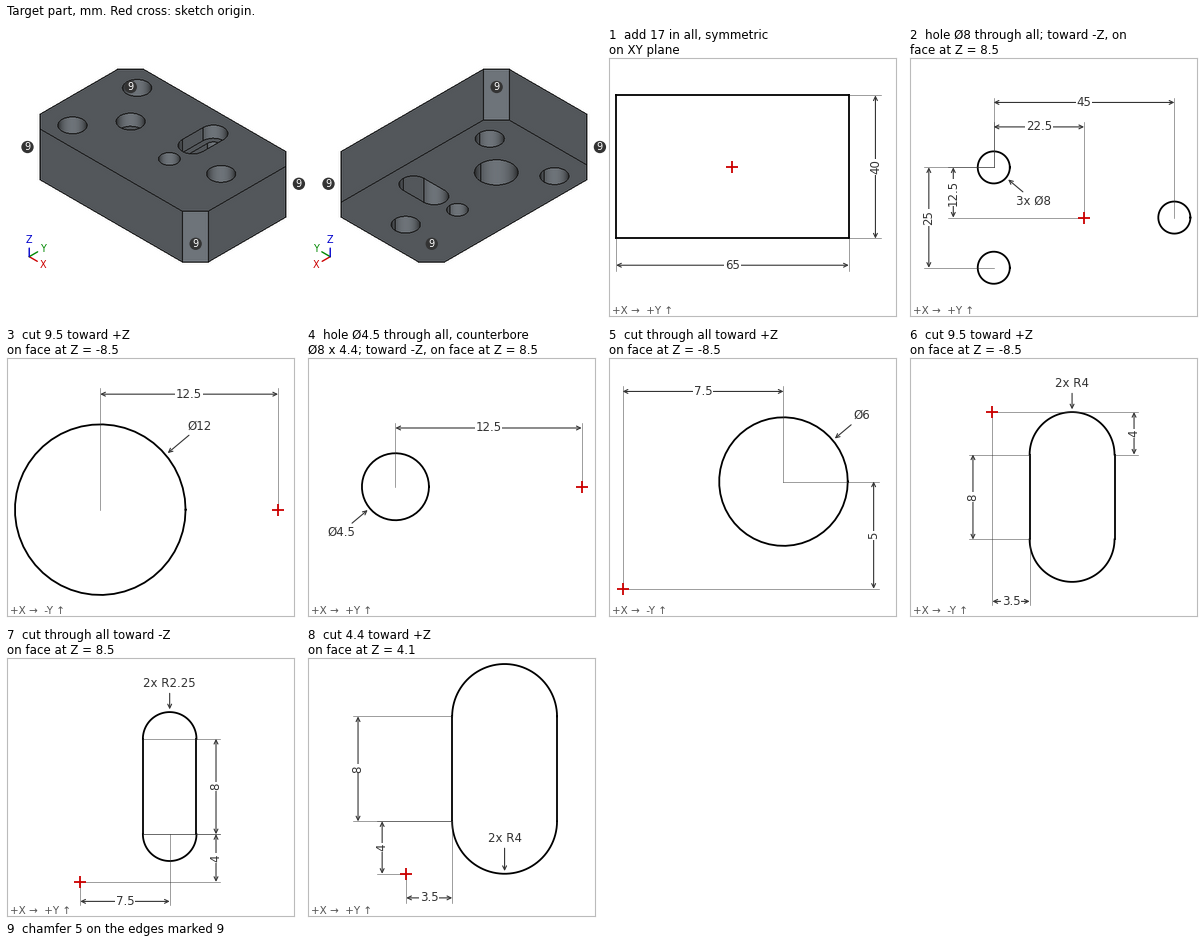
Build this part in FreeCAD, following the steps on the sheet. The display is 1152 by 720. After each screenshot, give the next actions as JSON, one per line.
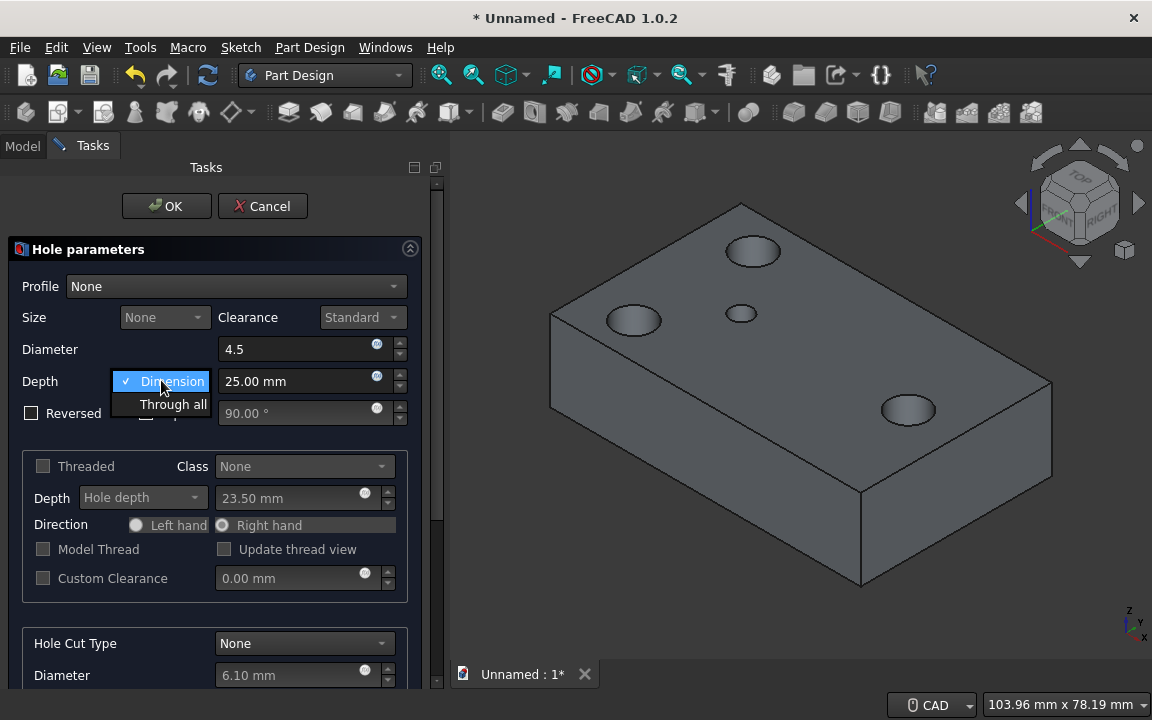
{"action": "left_click", "coordinate": [160, 404]}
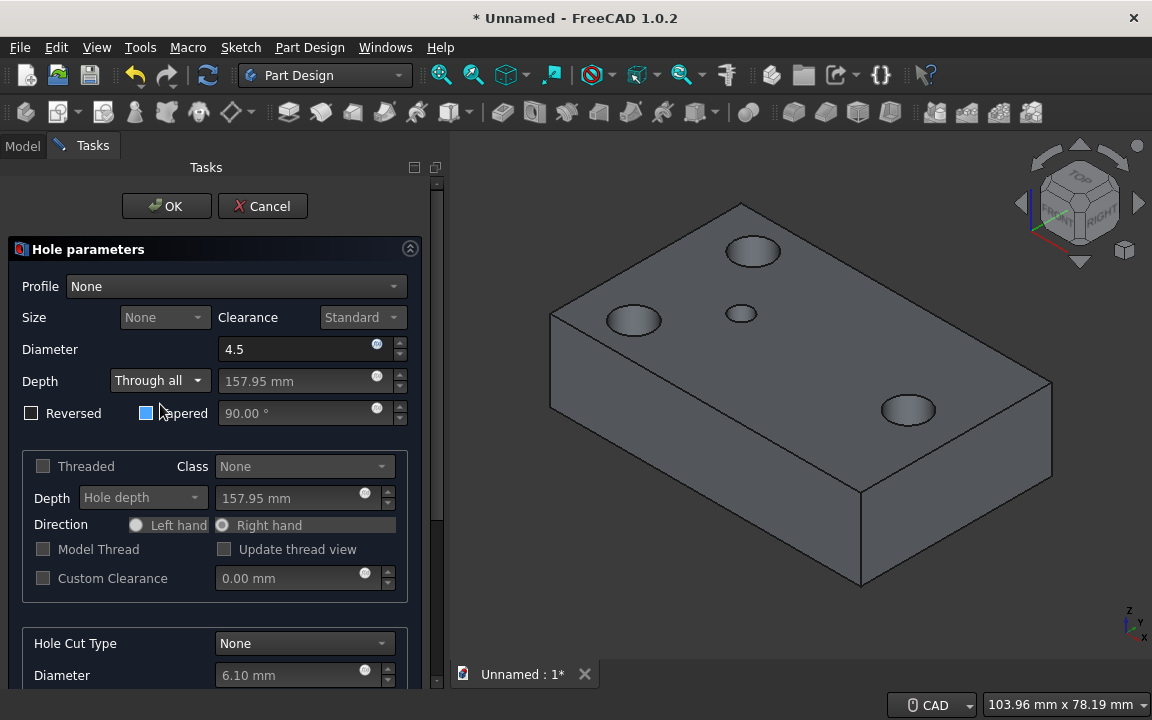
{"action": "left_click", "coordinate": [306, 644]}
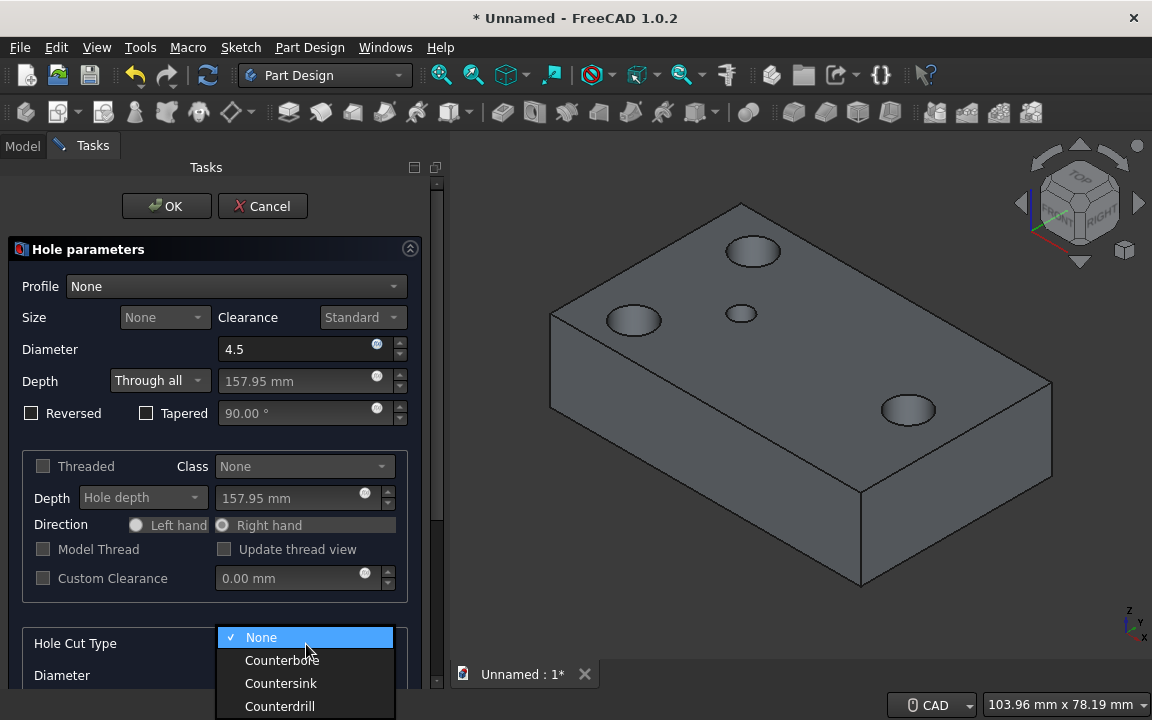
{"action": "left_click", "coordinate": [304, 660]}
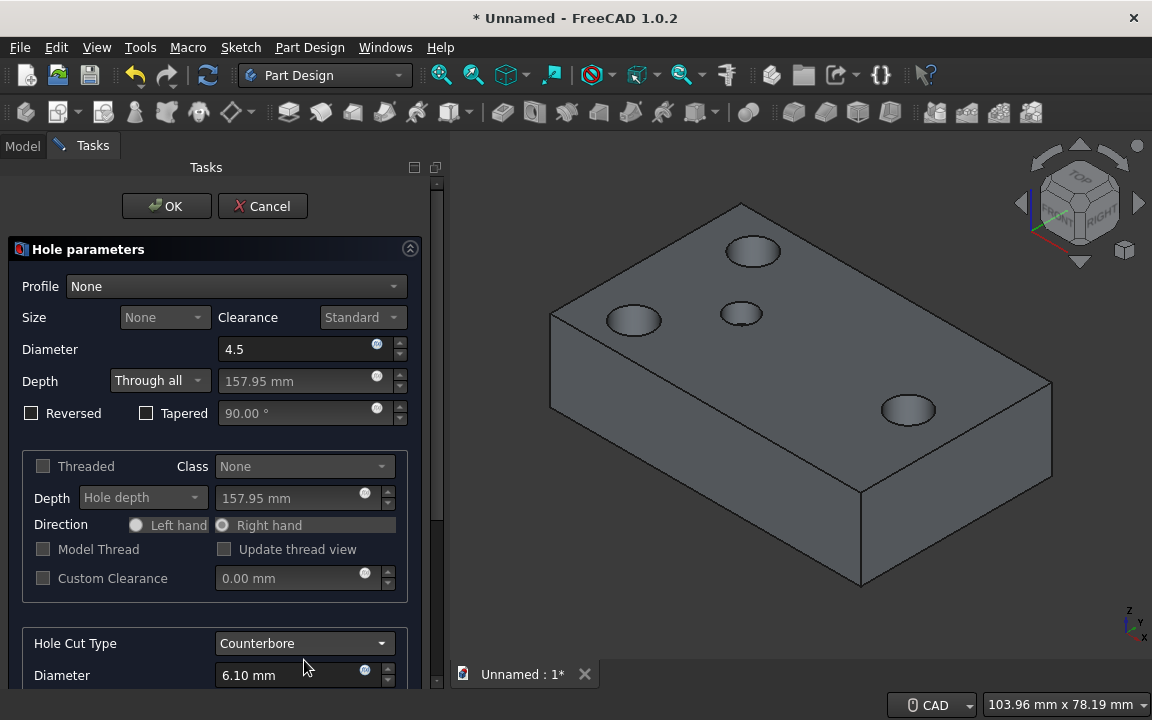
{"action": "triple_click", "coordinate": [298, 675]}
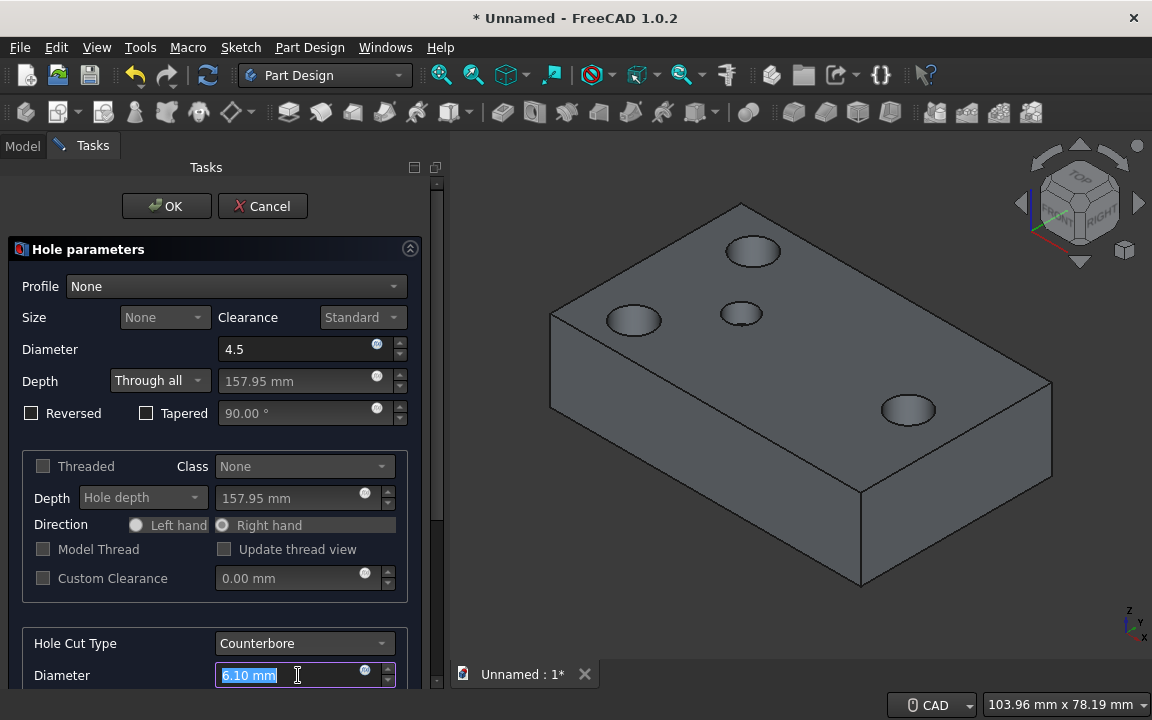
{"action": "type", "text": "8"}
{"action": "key", "text": "Tab"}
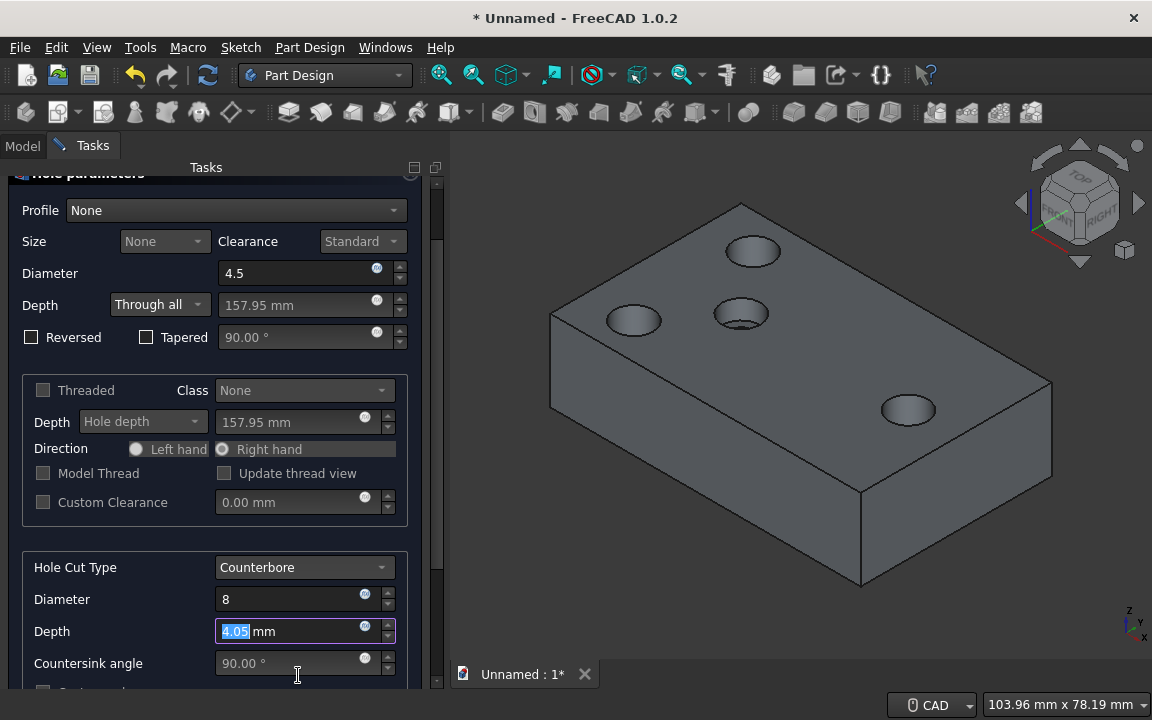
{"action": "type", "text": "4.4"}
{"action": "key", "text": "Tab"}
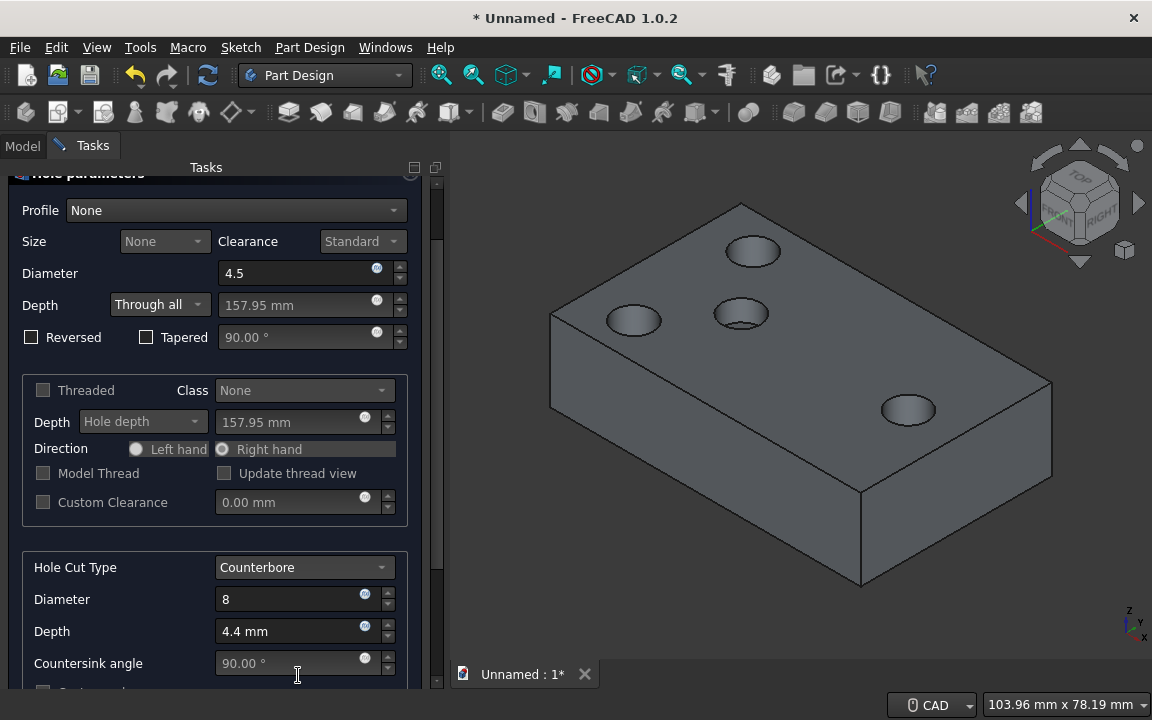
{"action": "scroll", "coordinate": [437, 432], "scroll_direction": "up", "scroll_amount": 3}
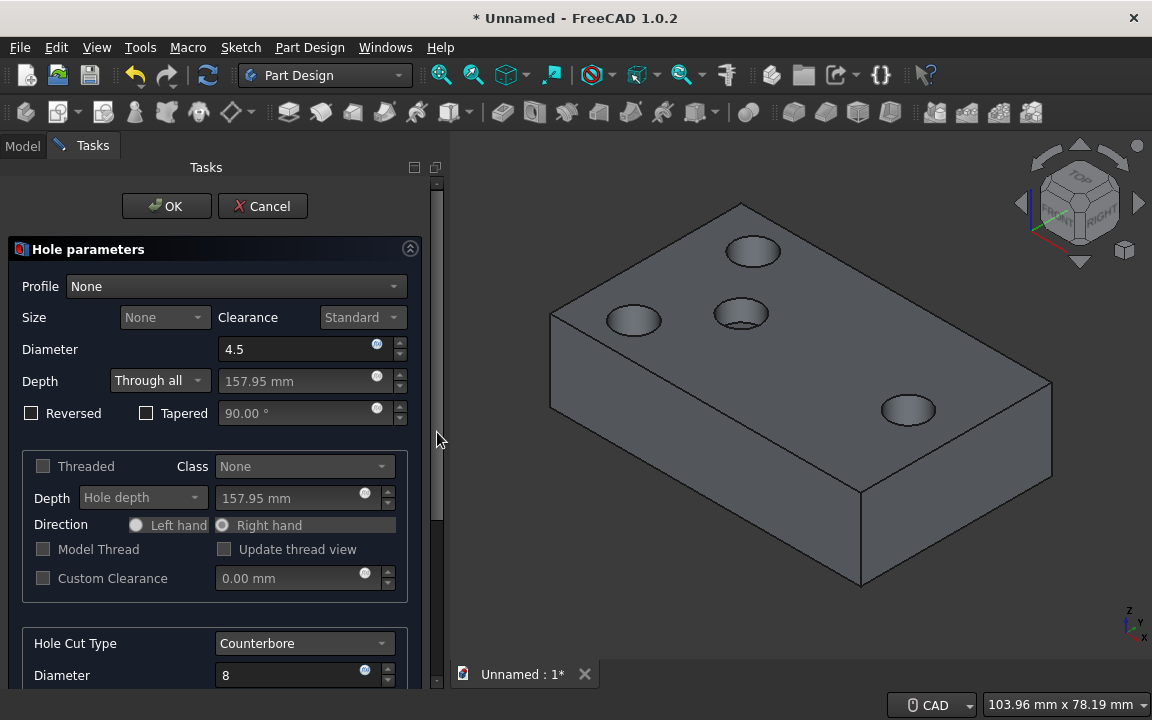
{"action": "left_click", "coordinate": [167, 206]}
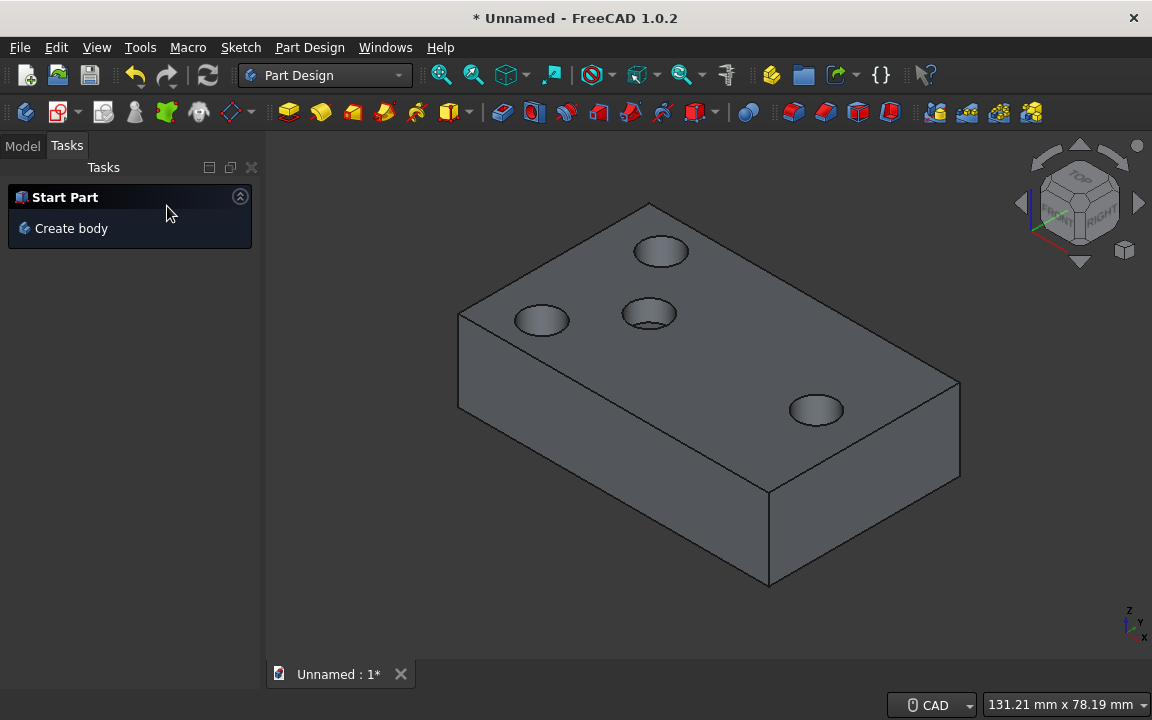
{"action": "key", "text": "5"}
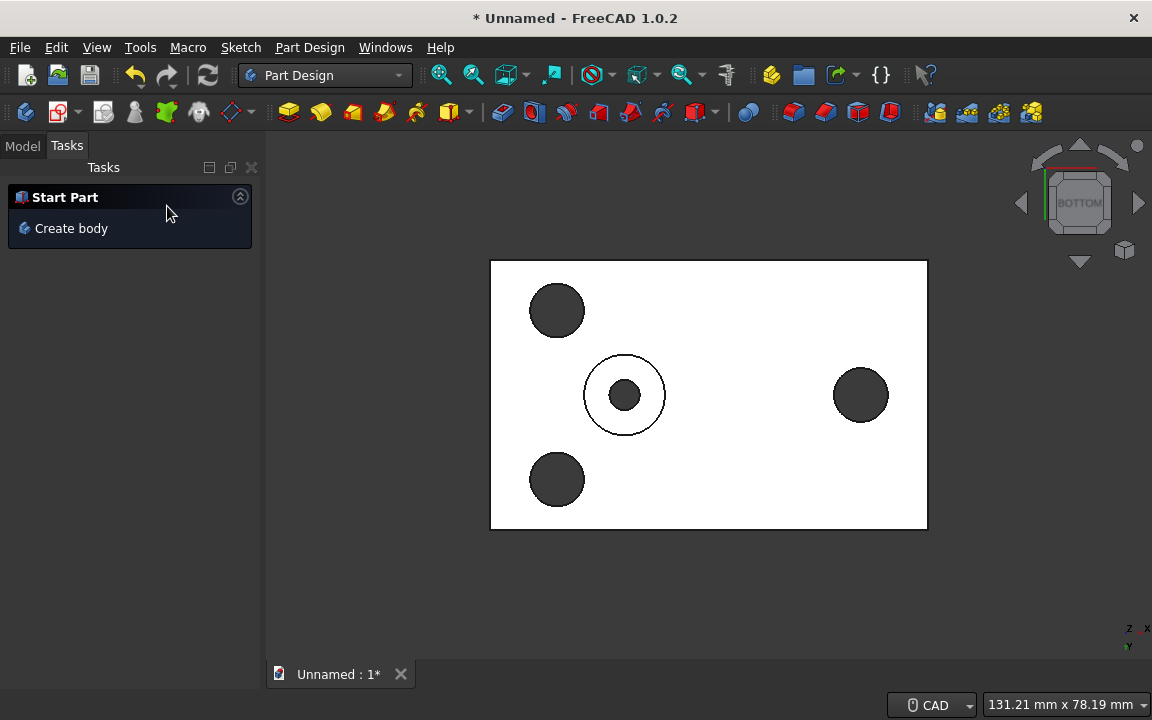
{"action": "left_click", "coordinate": [772, 355]}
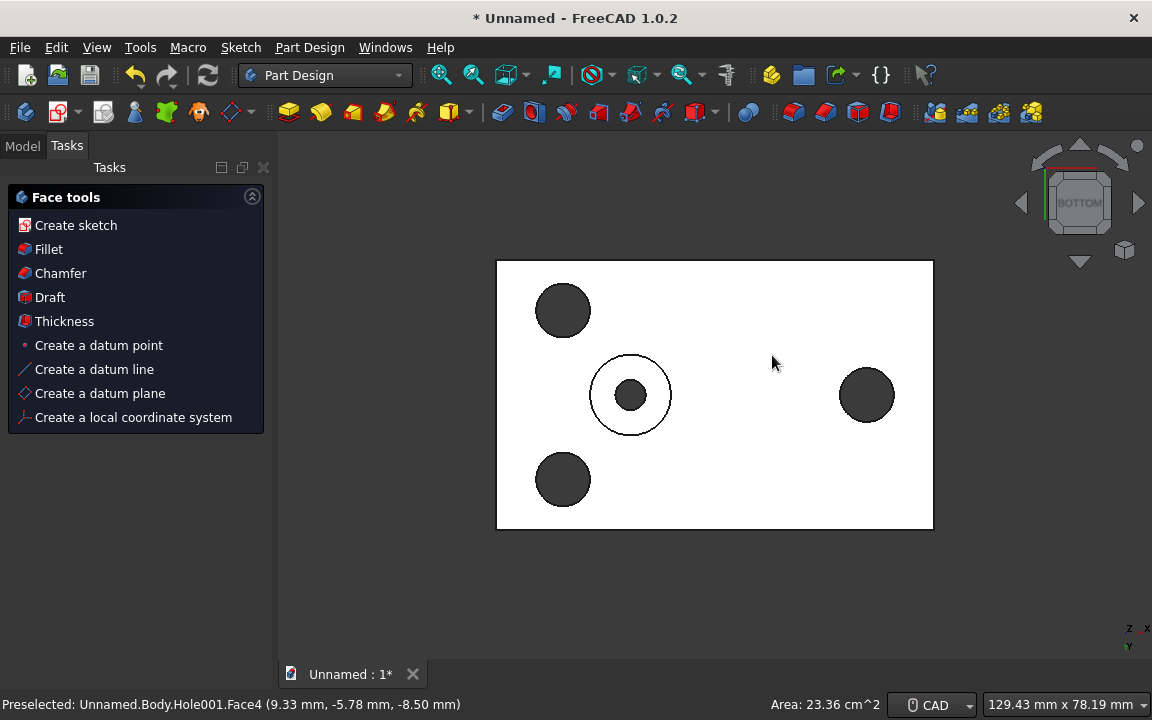
{"action": "left_click", "coordinate": [58, 112]}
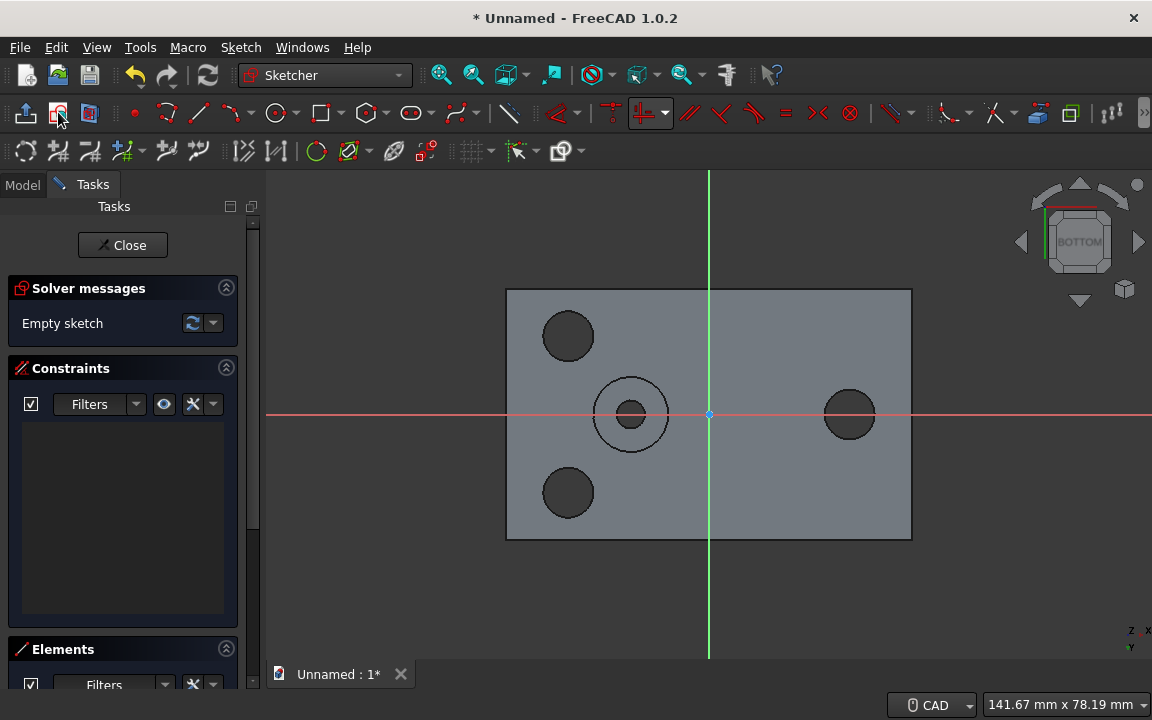
{"action": "scroll", "coordinate": [762, 385], "scroll_direction": "up", "scroll_amount": 9}